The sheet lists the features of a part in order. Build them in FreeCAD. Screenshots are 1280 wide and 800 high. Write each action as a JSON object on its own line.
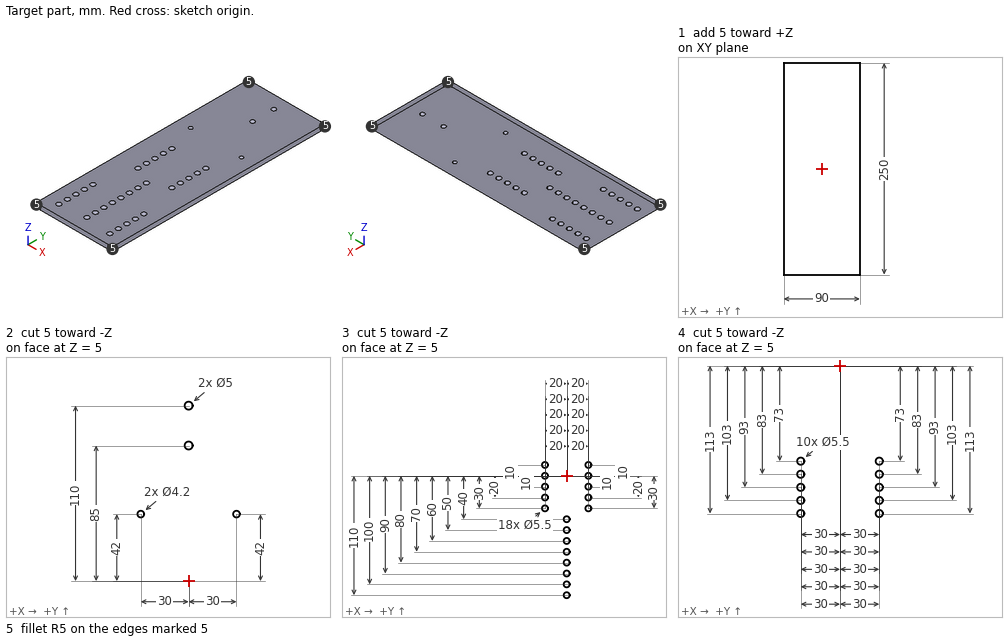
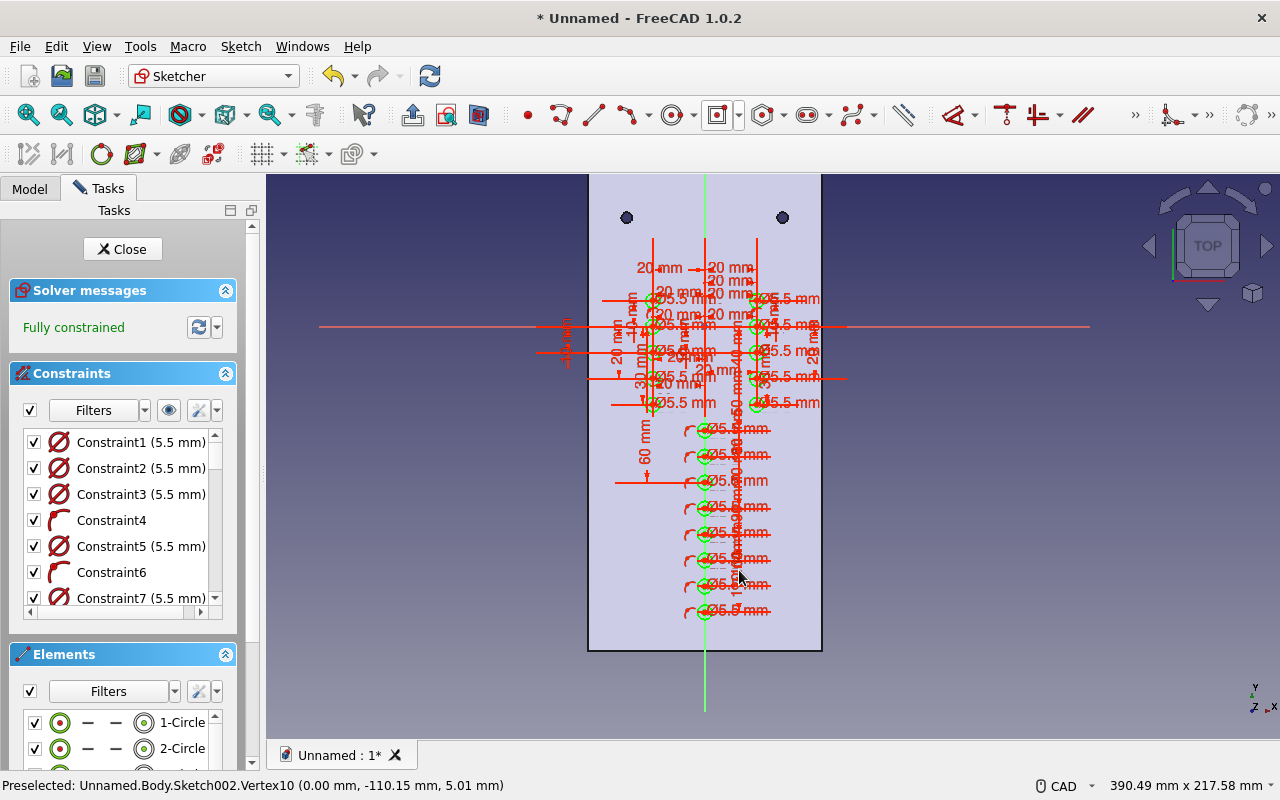
{"action": "left_click", "coordinate": [123, 249]}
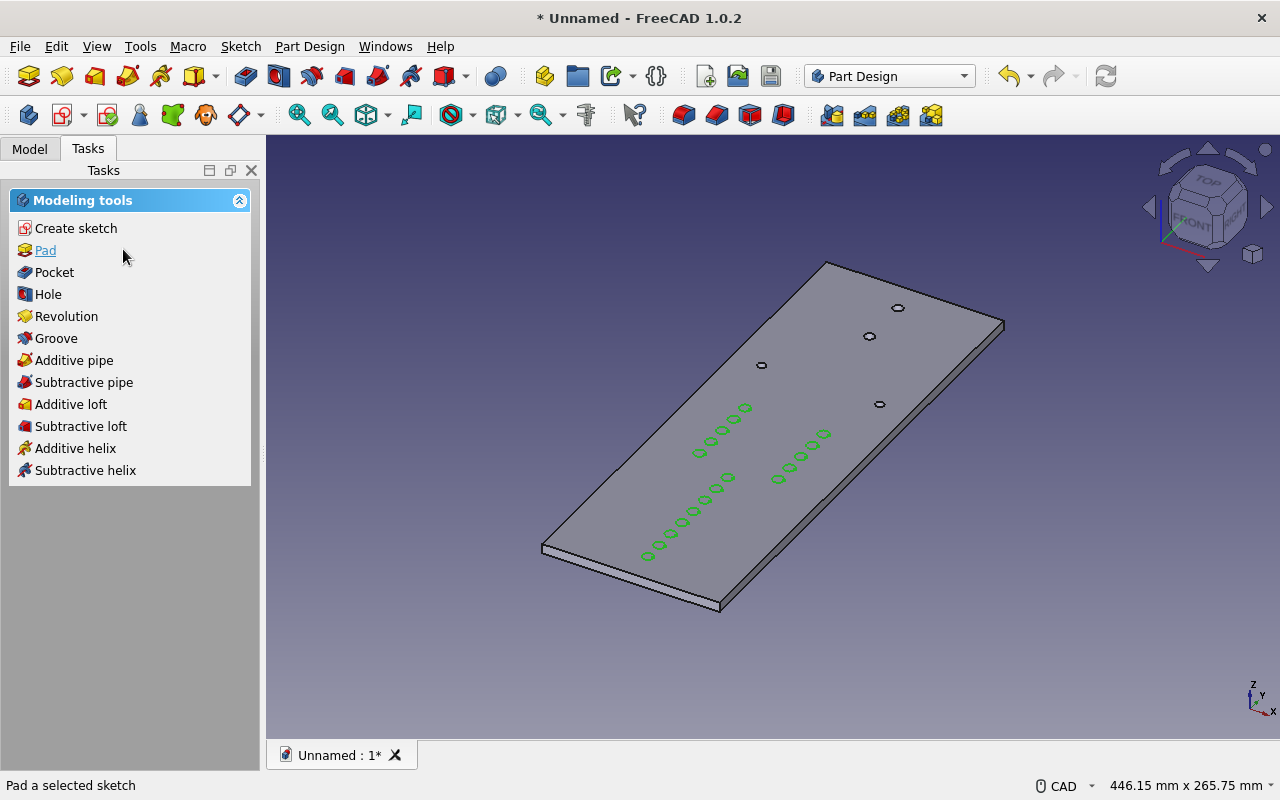
{"action": "left_click", "coordinate": [246, 76]}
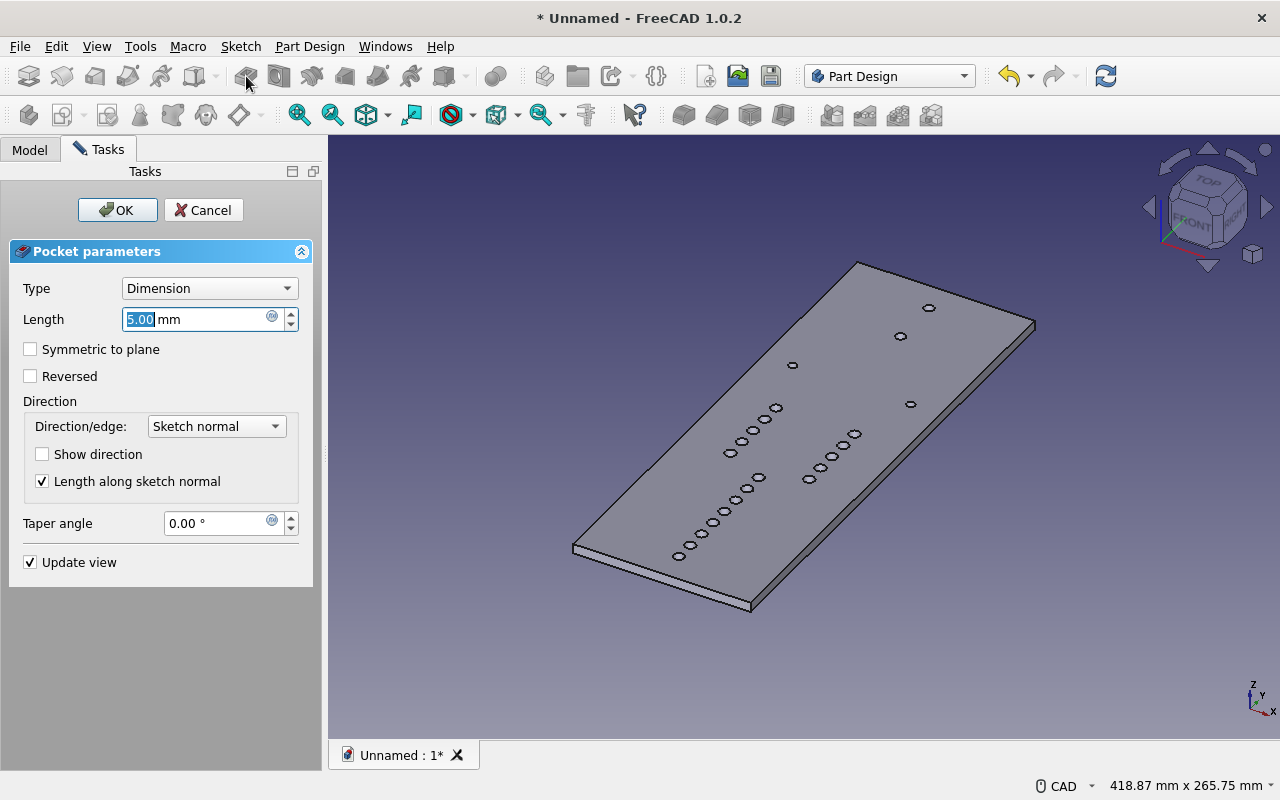
{"action": "type", "text": "5"}
{"action": "key", "text": "Tab"}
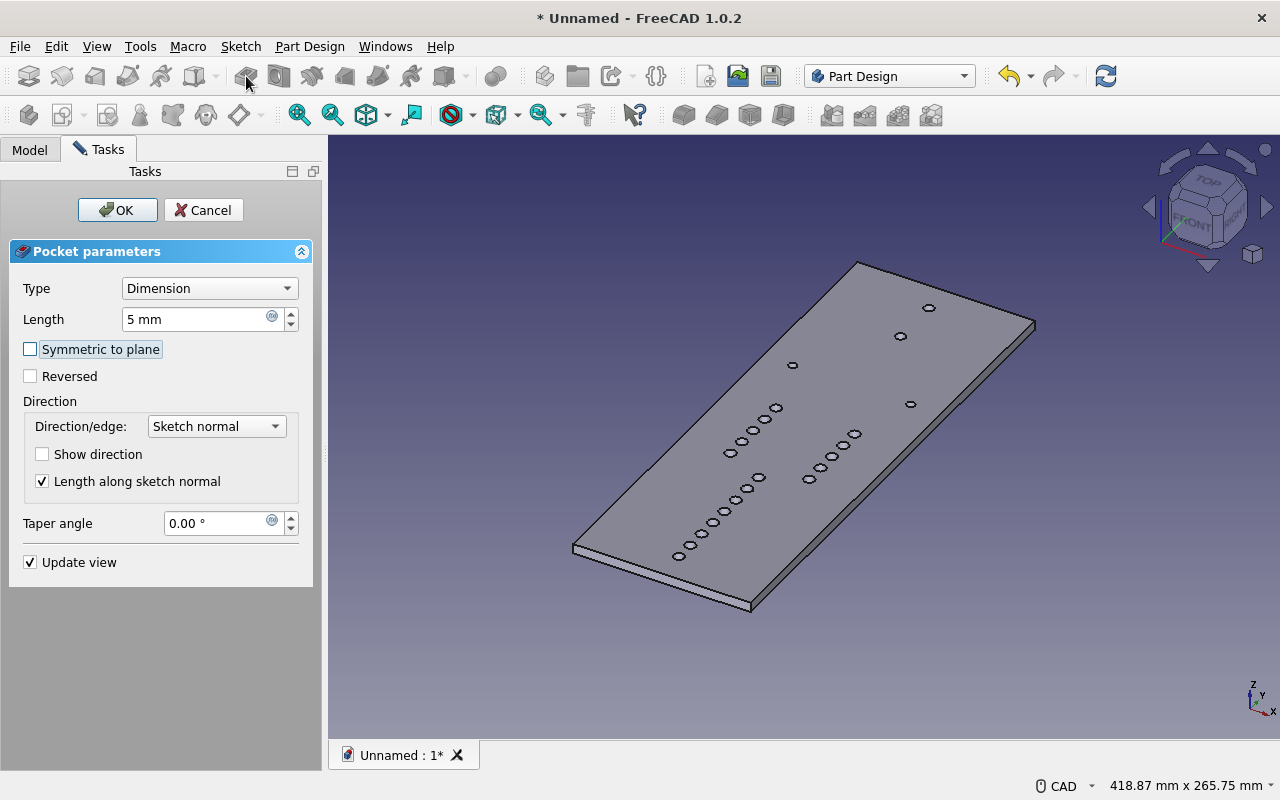
{"action": "left_click", "coordinate": [118, 210]}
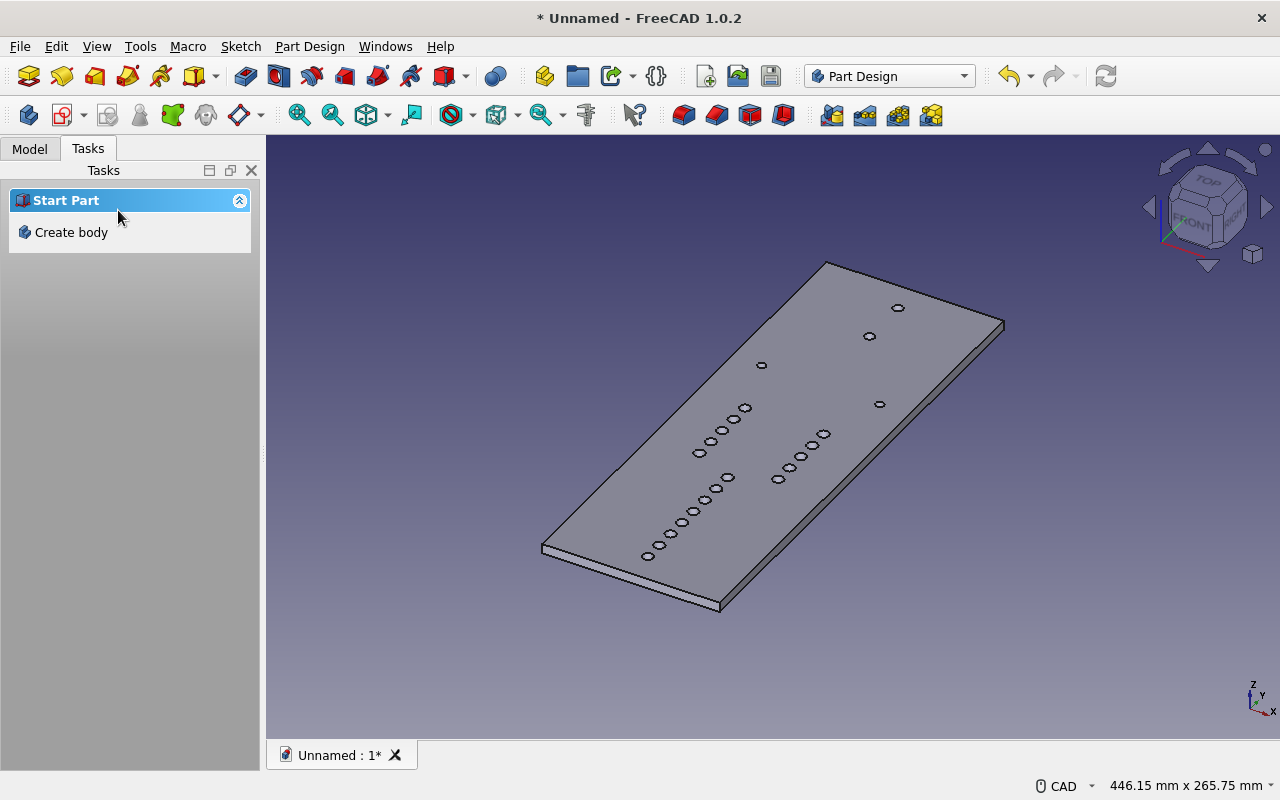
{"action": "left_click", "coordinate": [814, 391]}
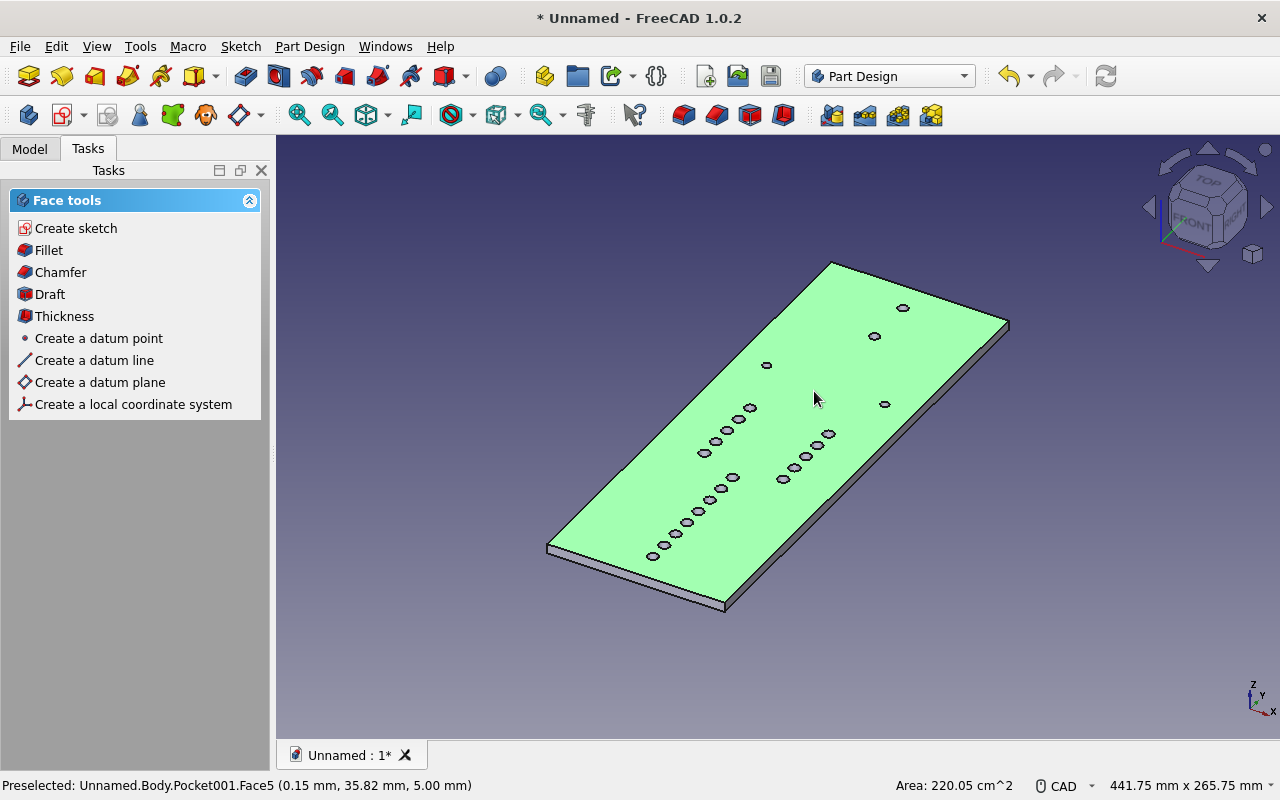
{"action": "left_click", "coordinate": [62, 116]}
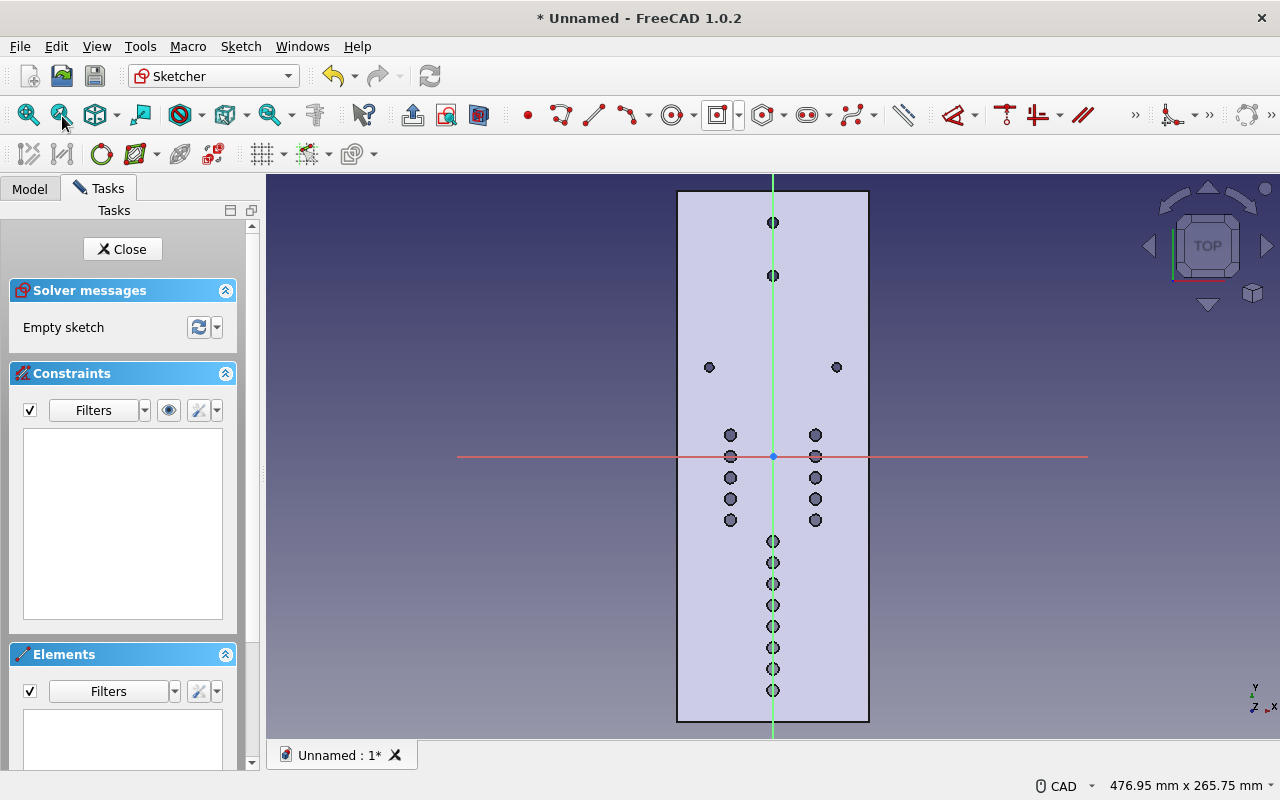
{"action": "scroll", "coordinate": [395, 202], "scroll_direction": "down", "scroll_amount": 1}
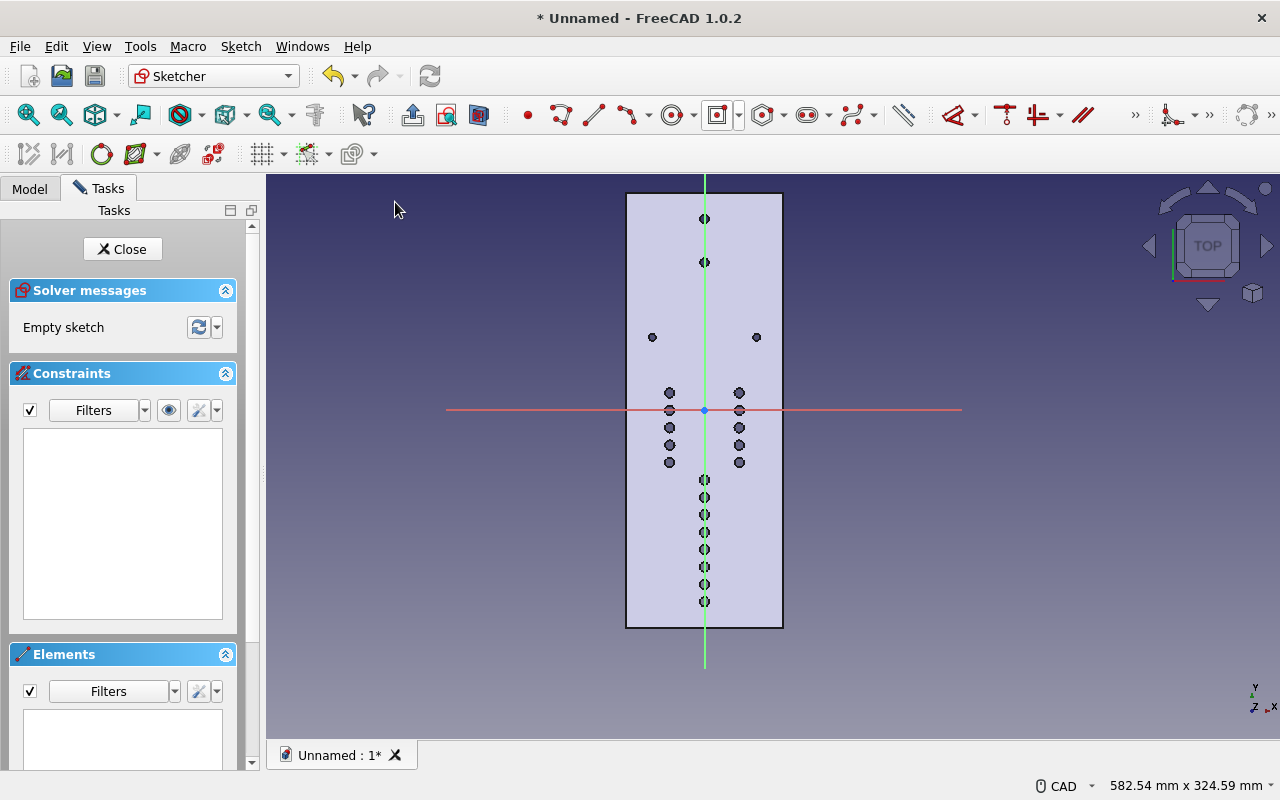
{"action": "scroll", "coordinate": [705, 578], "scroll_direction": "up", "scroll_amount": 3}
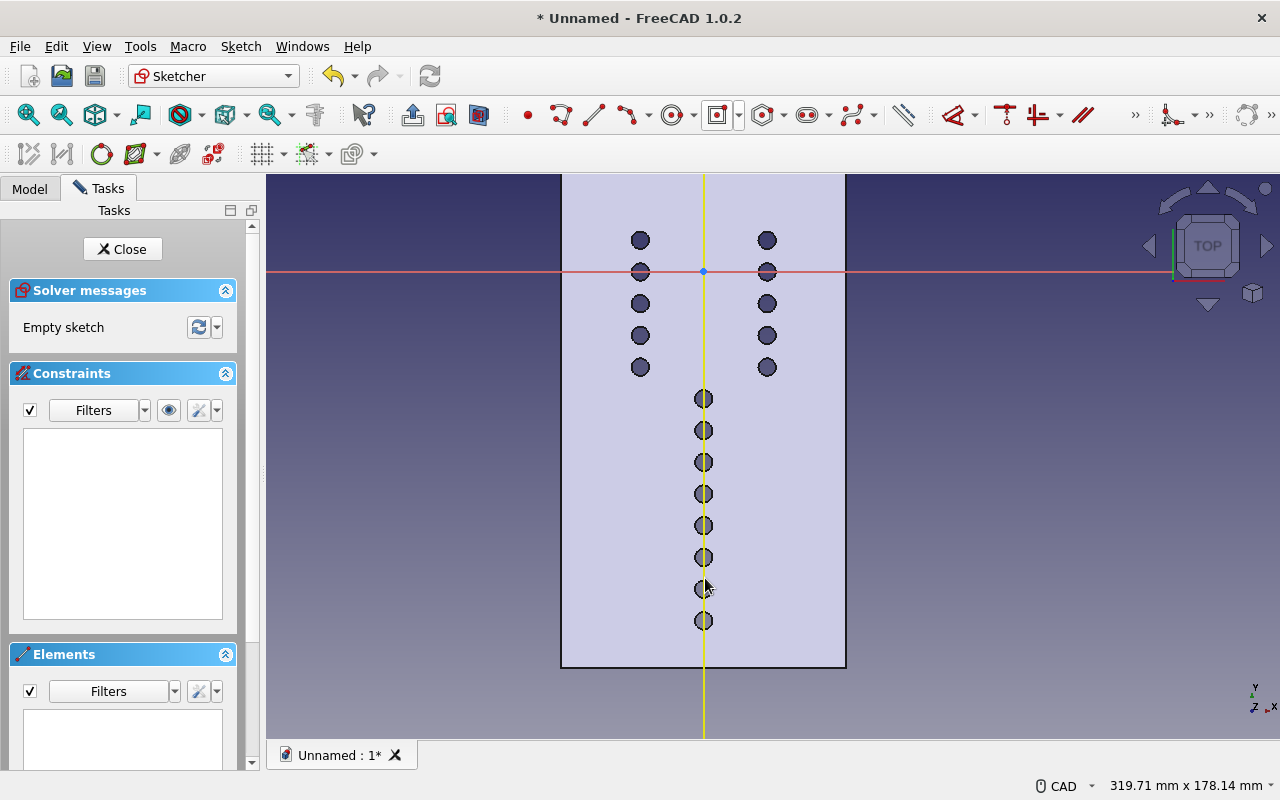
{"action": "key", "text": "g c"}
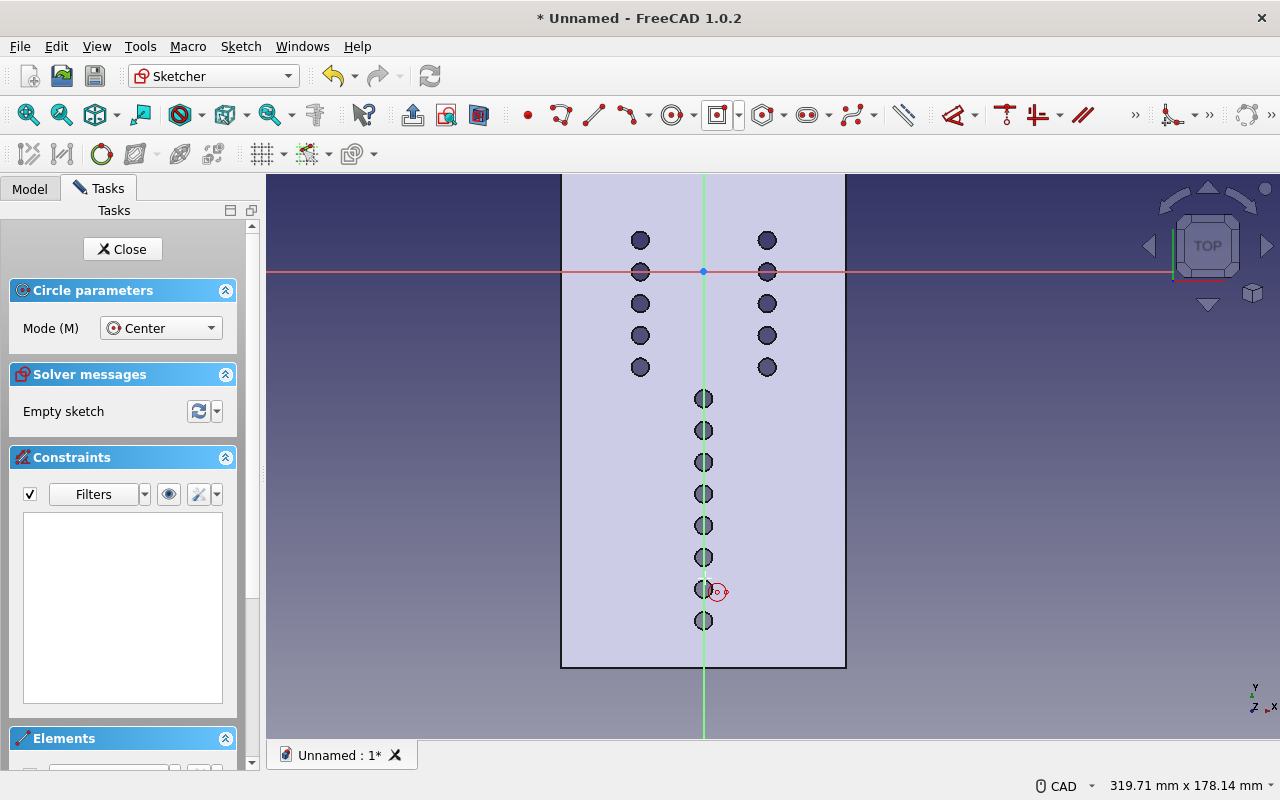
{"action": "scroll", "coordinate": [609, 630], "scroll_direction": "up", "scroll_amount": 5}